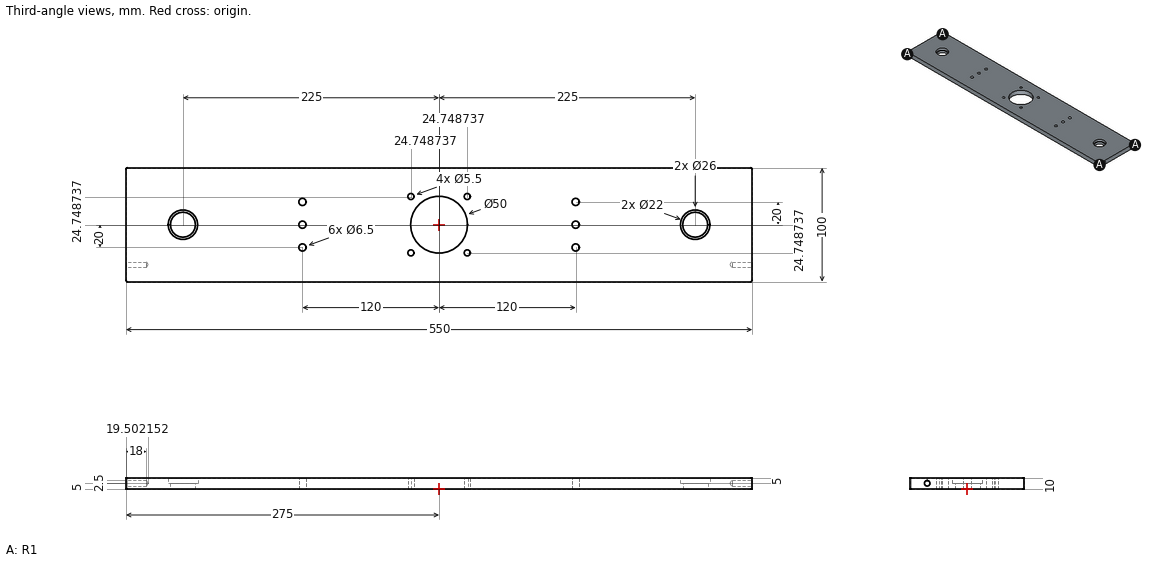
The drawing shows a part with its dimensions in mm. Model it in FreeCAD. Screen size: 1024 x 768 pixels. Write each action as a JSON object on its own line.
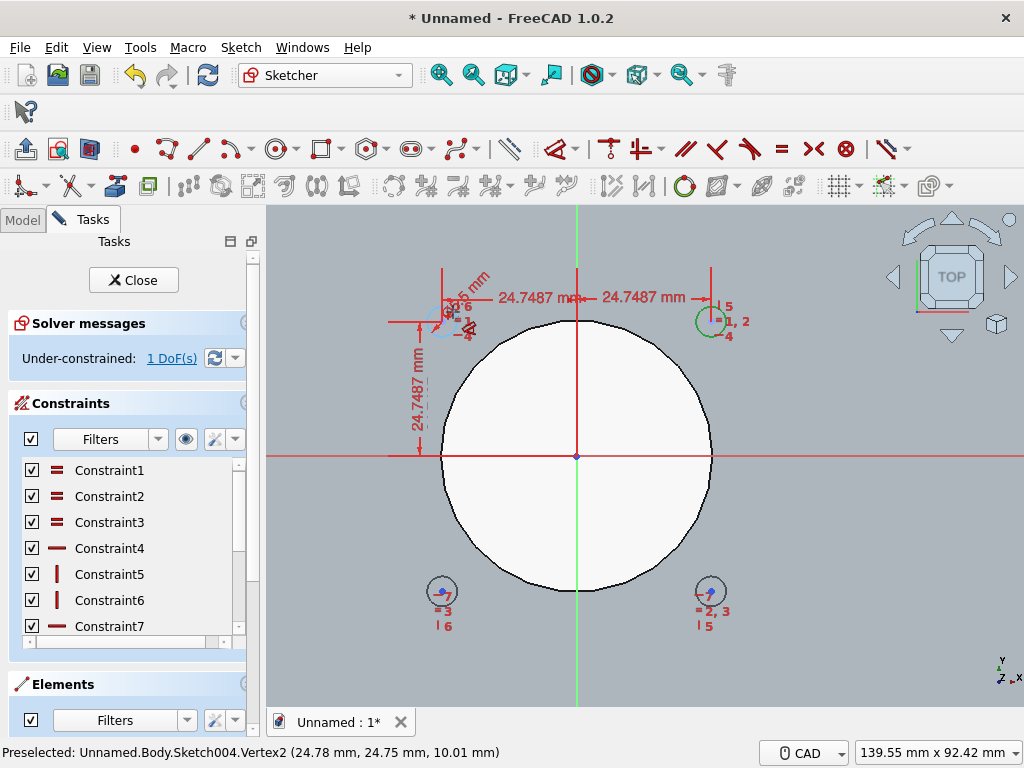
{"action": "left_click", "coordinate": [711, 591]}
{"action": "left_click", "coordinate": [745, 524]}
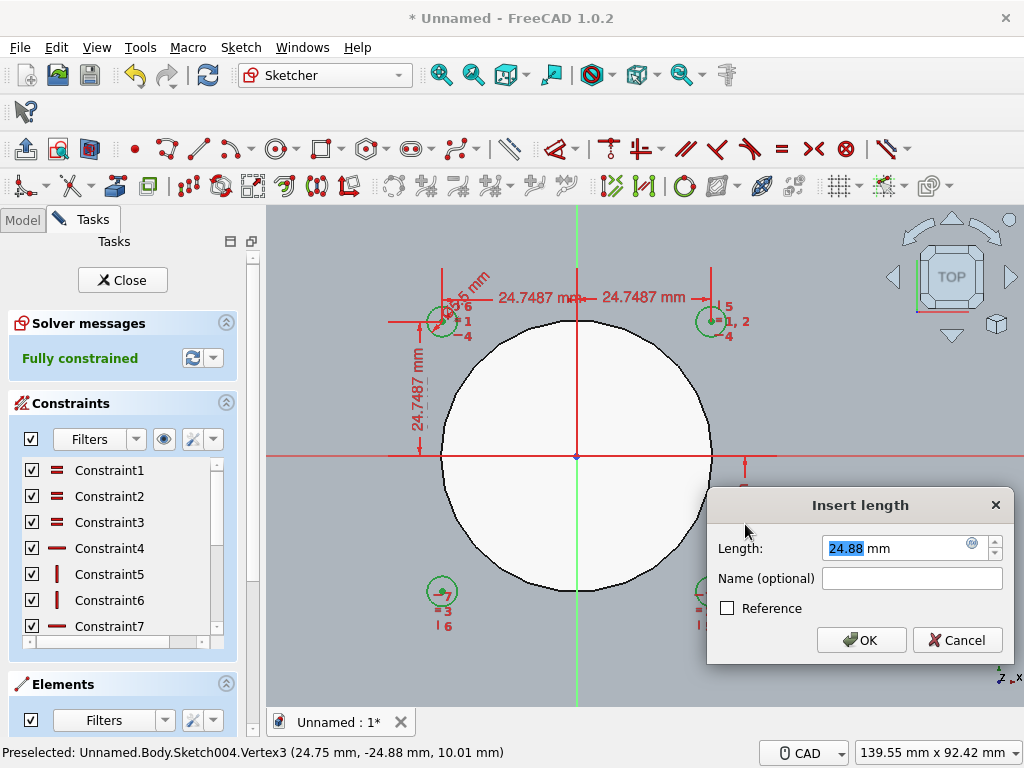
{"action": "type", "text": "24.748737"}
{"action": "key", "text": "Return"}
{"action": "key", "text": "Escape"}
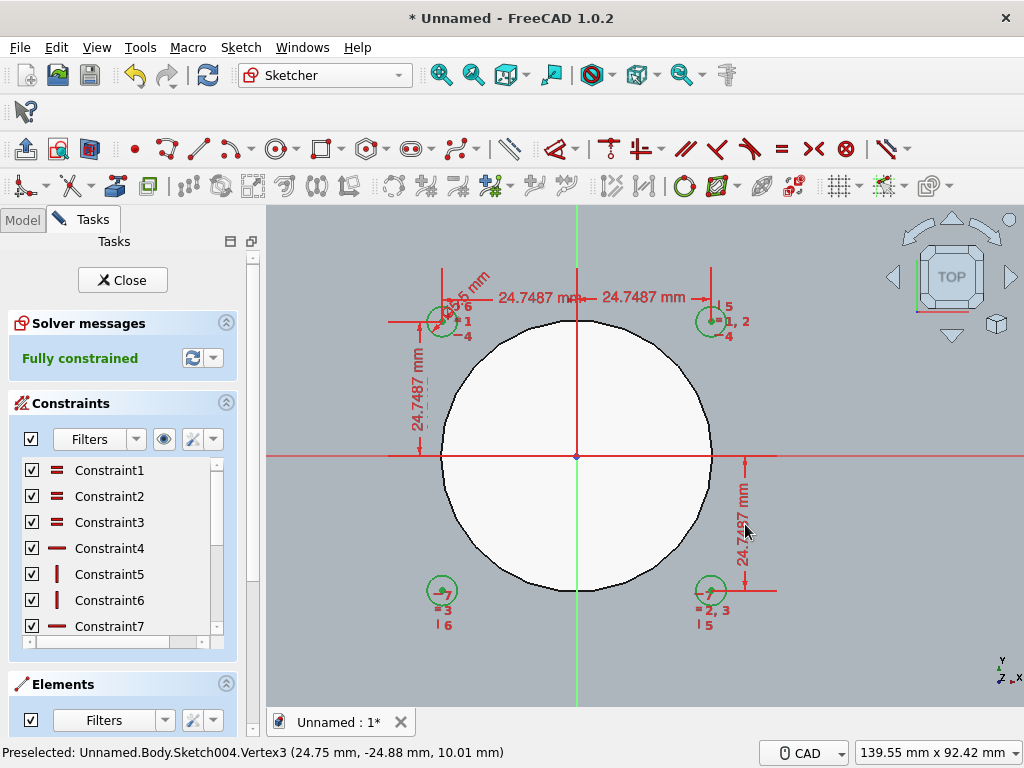
{"action": "left_click", "coordinate": [123, 280]}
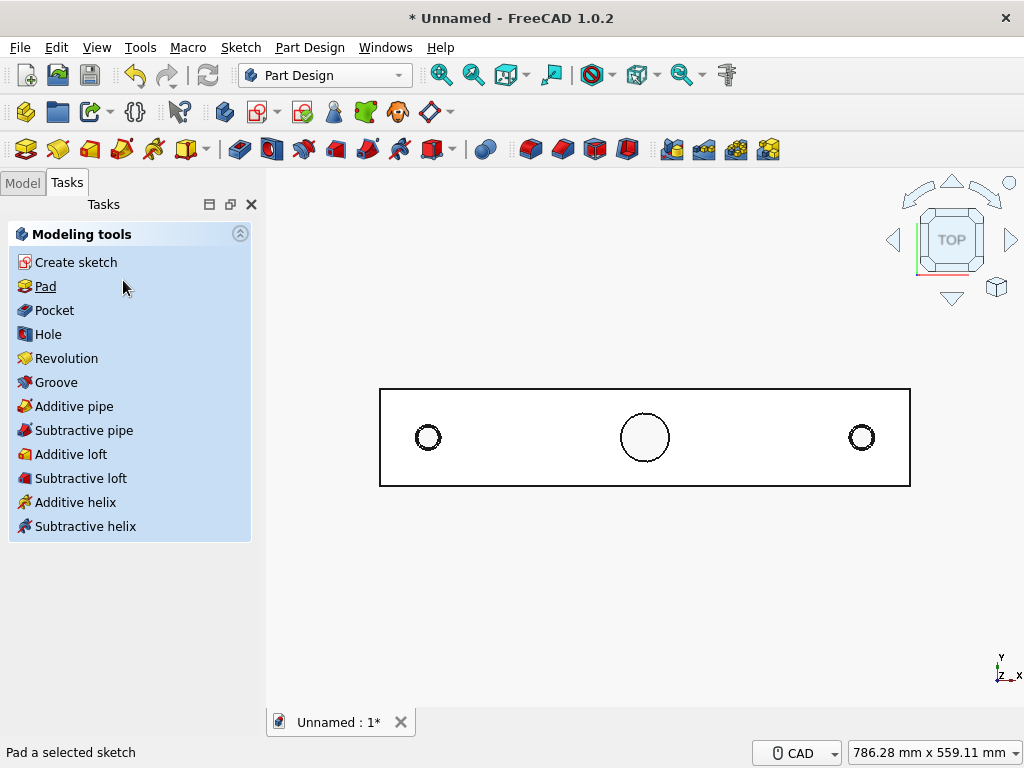
{"action": "left_click", "coordinate": [240, 150]}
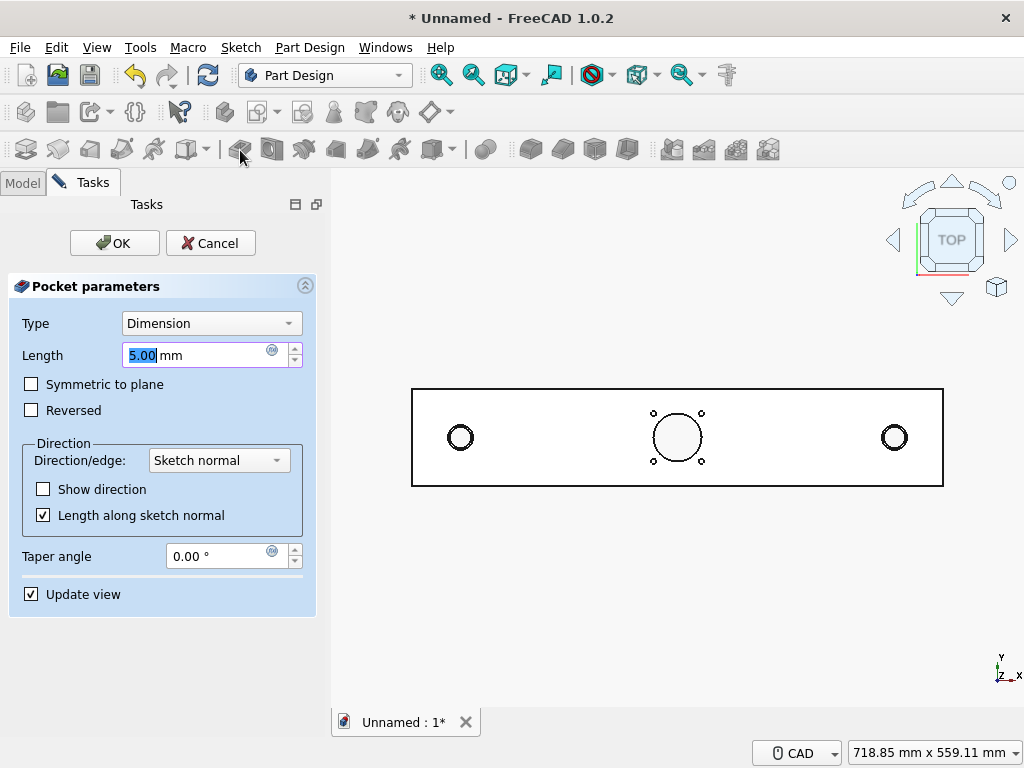
{"action": "left_click", "coordinate": [212, 324]}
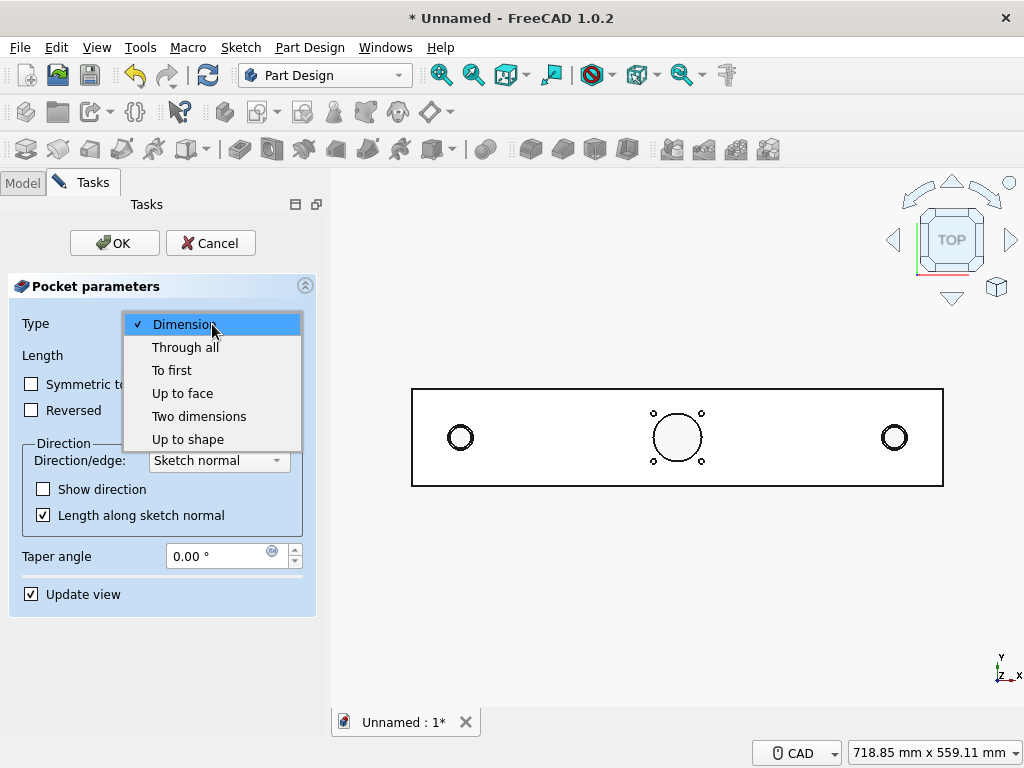
{"action": "left_click", "coordinate": [212, 348]}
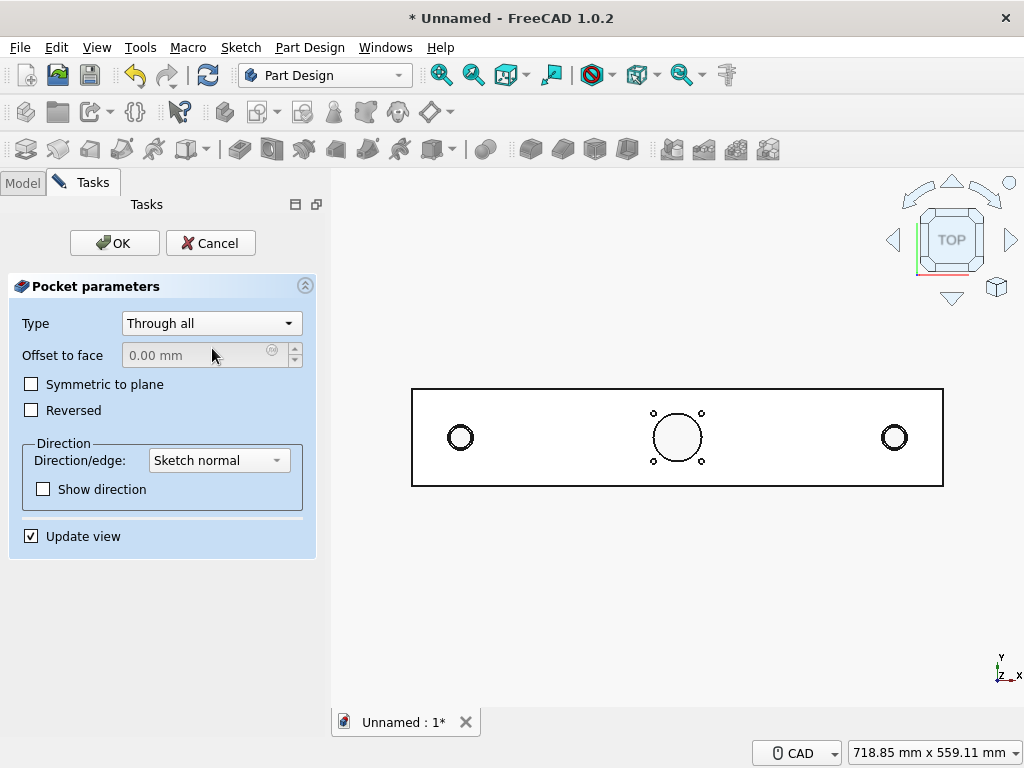
{"action": "left_click", "coordinate": [115, 243]}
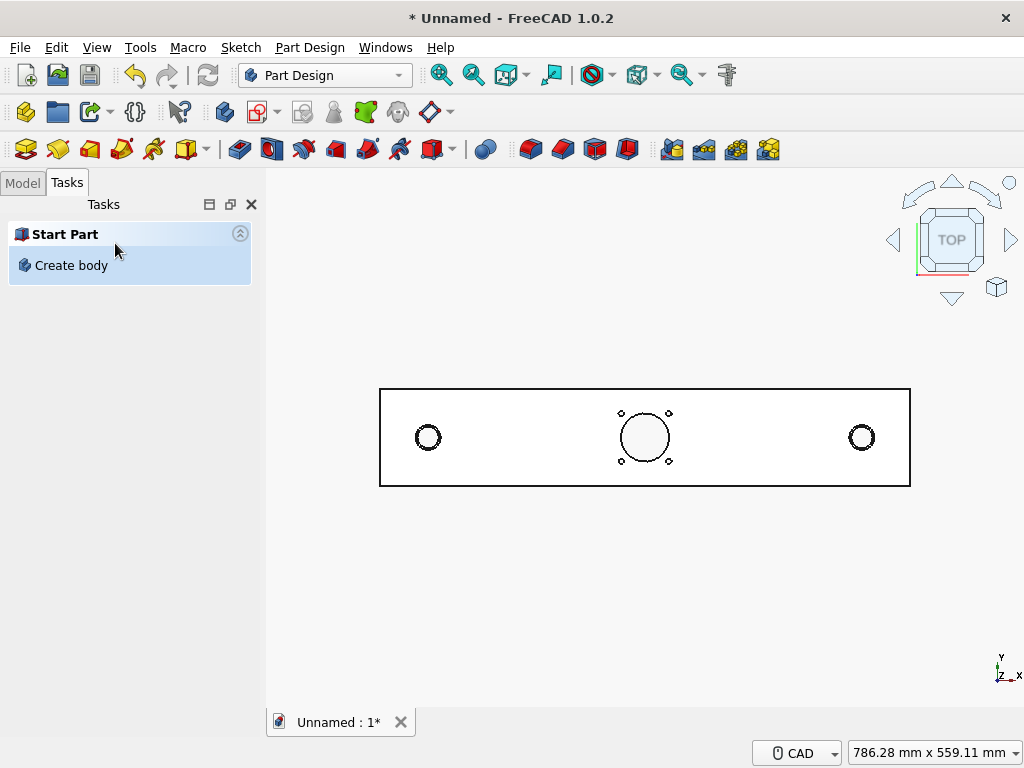
{"action": "left_click", "coordinate": [796, 437]}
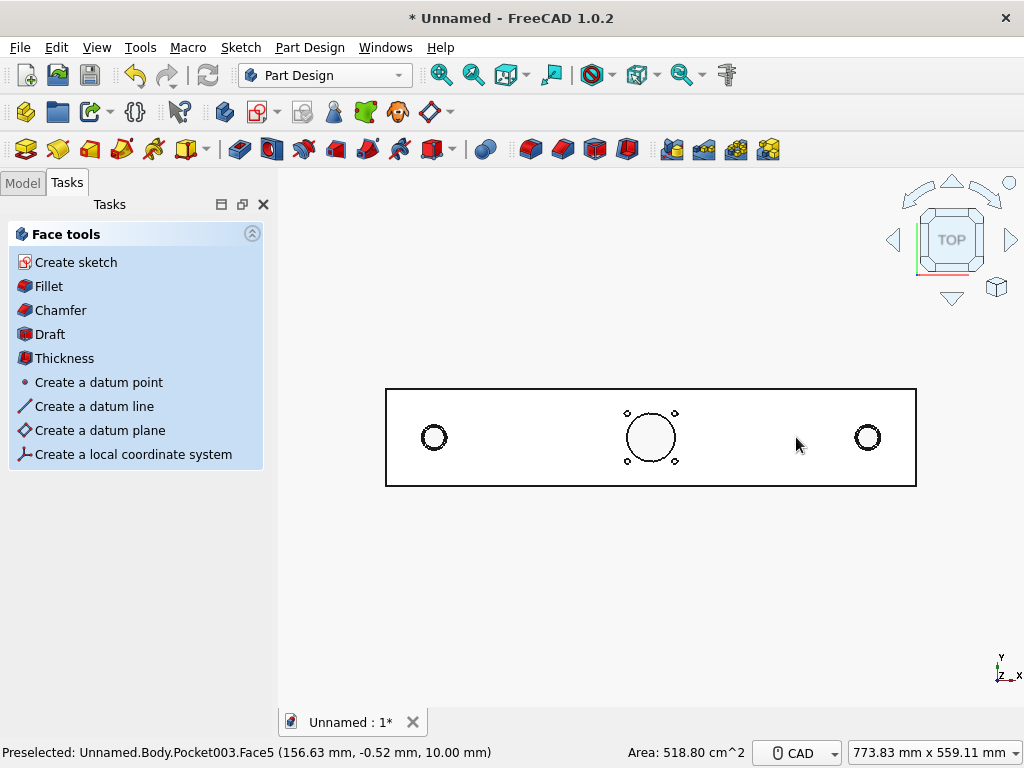
{"action": "left_click", "coordinate": [258, 112]}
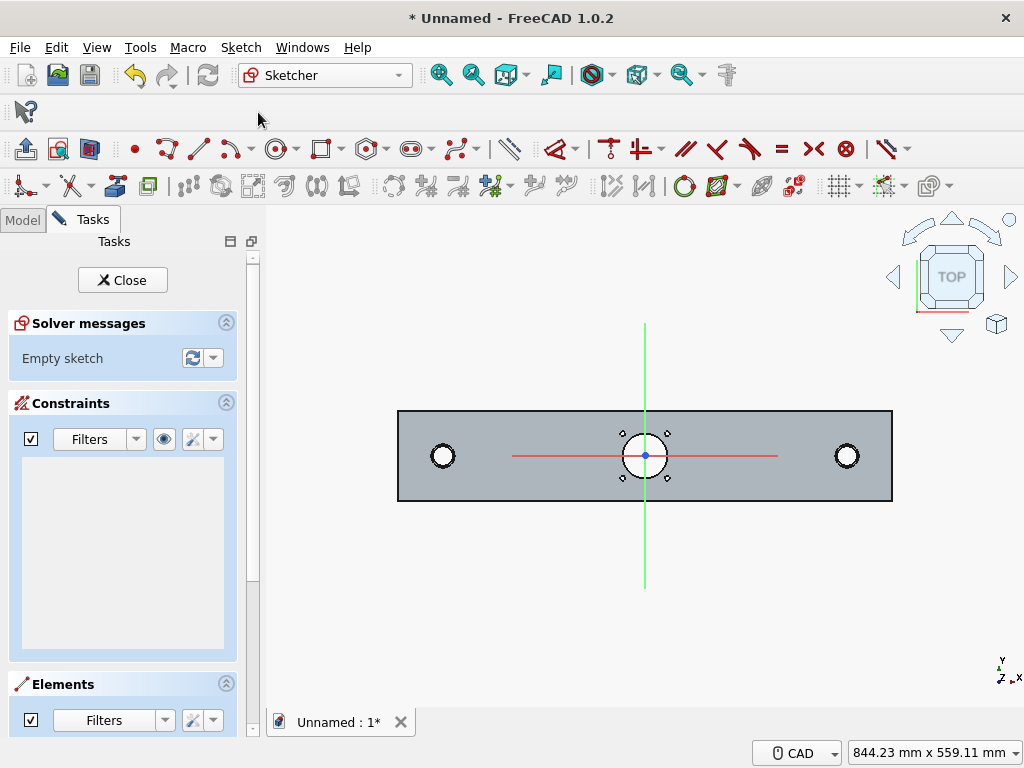
{"action": "scroll", "coordinate": [728, 456], "scroll_direction": "up", "scroll_amount": 3}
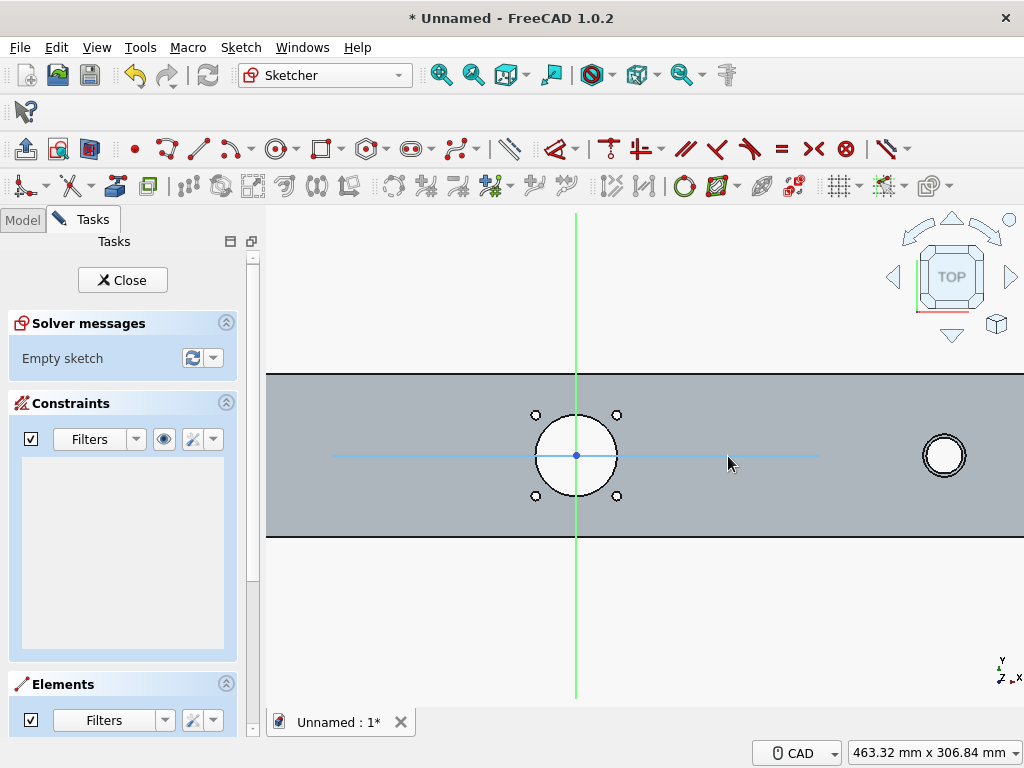
{"action": "left_click", "coordinate": [276, 150]}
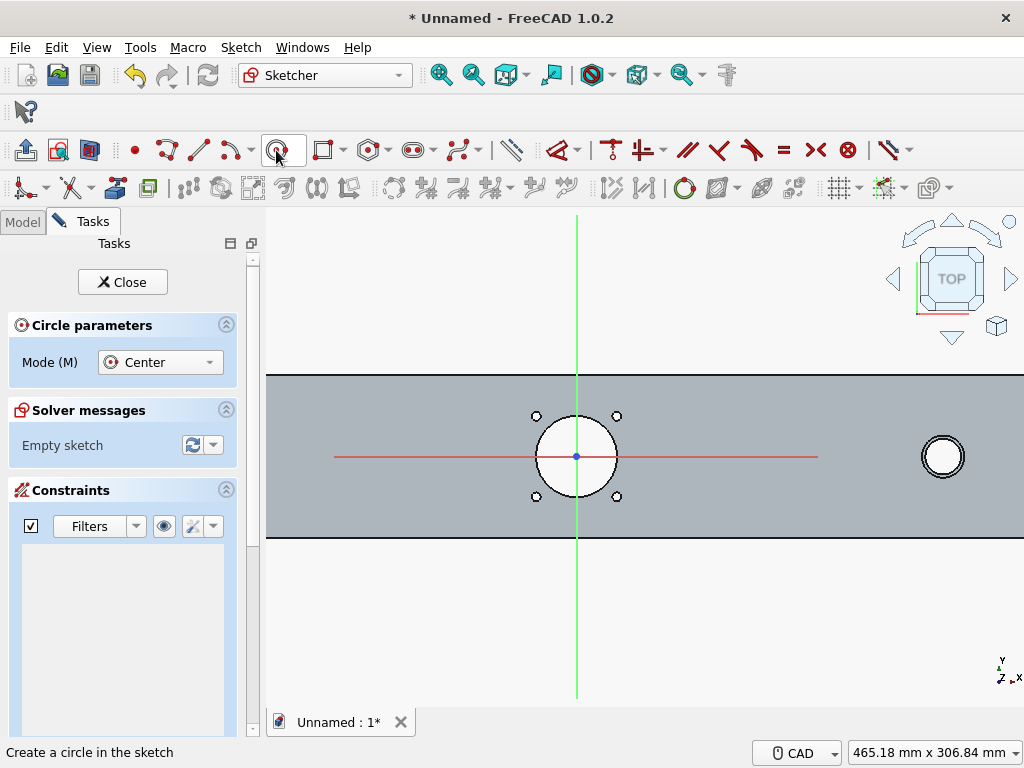
{"action": "scroll", "coordinate": [381, 489], "scroll_direction": "up", "scroll_amount": 8}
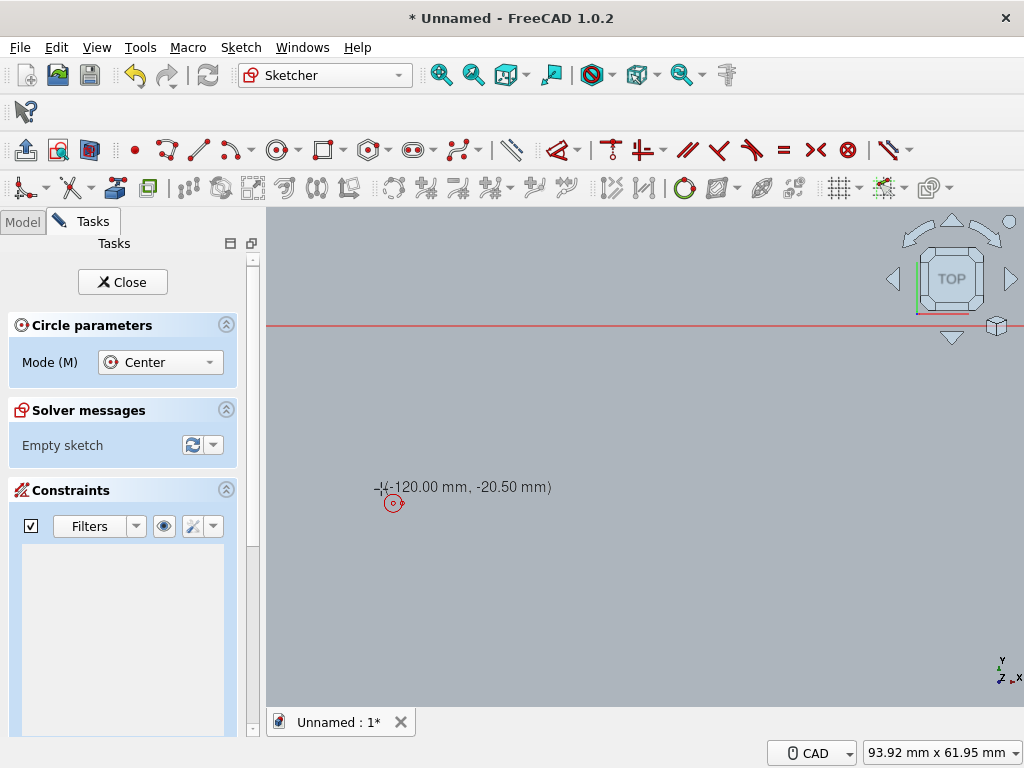
{"action": "scroll", "coordinate": [381, 490], "scroll_direction": "down", "scroll_amount": 8}